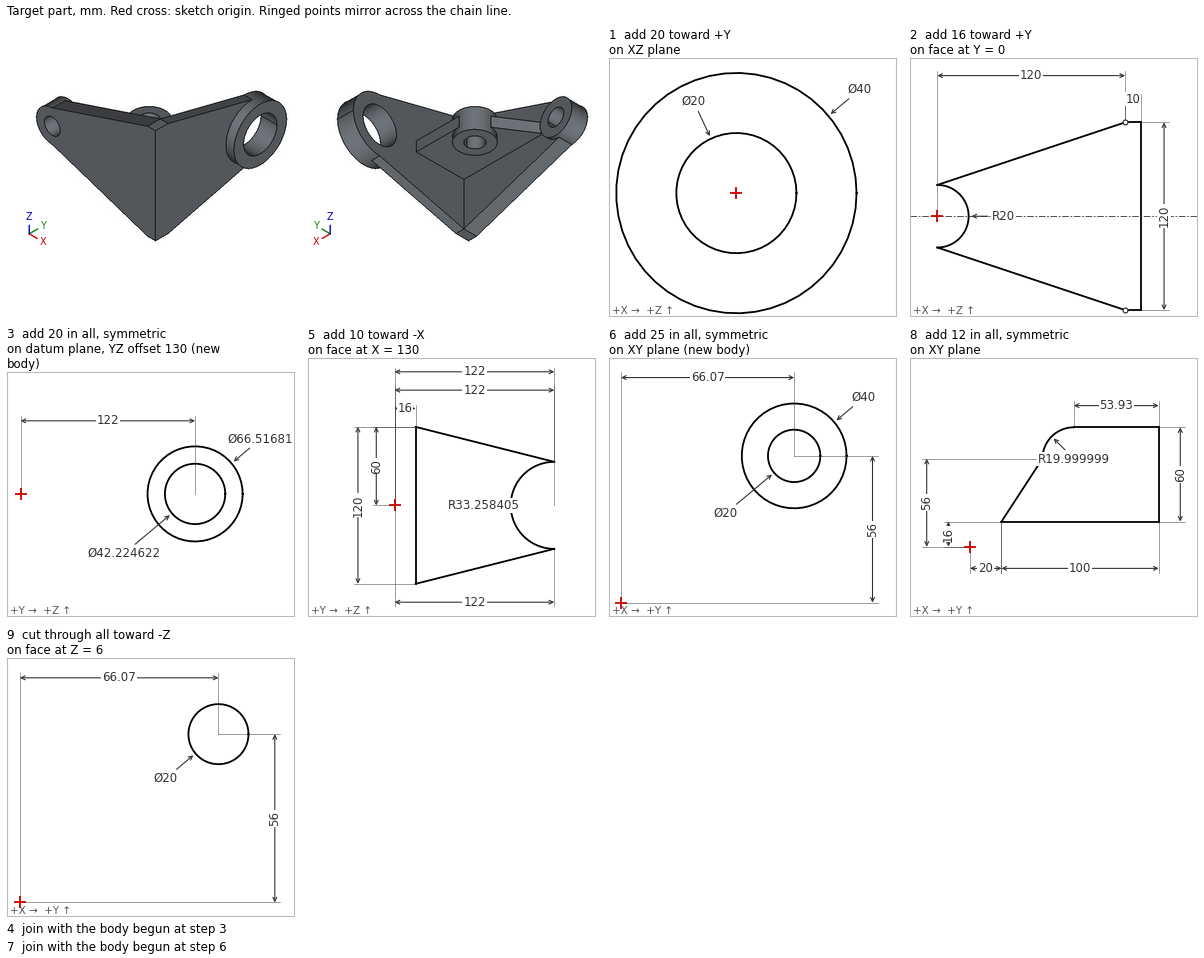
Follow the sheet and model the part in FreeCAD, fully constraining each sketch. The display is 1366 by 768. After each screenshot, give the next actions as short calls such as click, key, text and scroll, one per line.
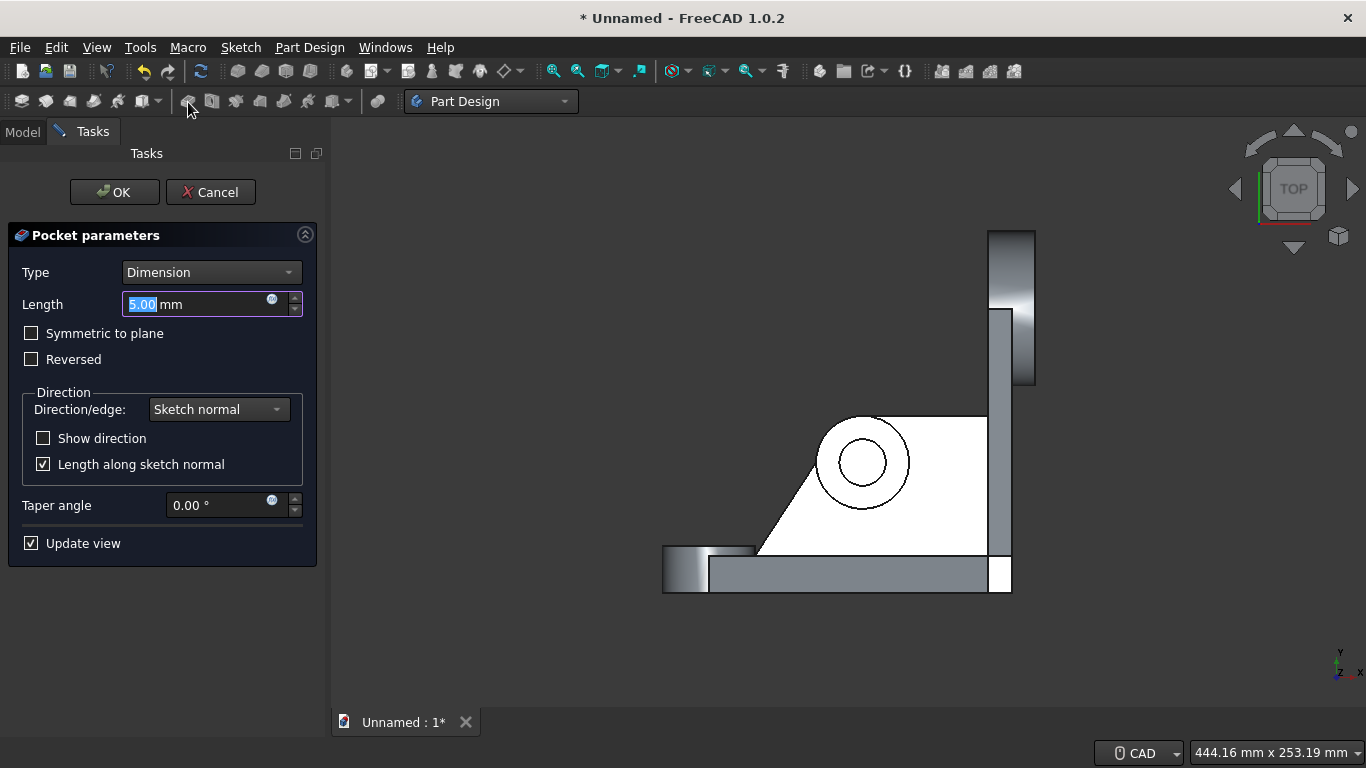
click(212, 272)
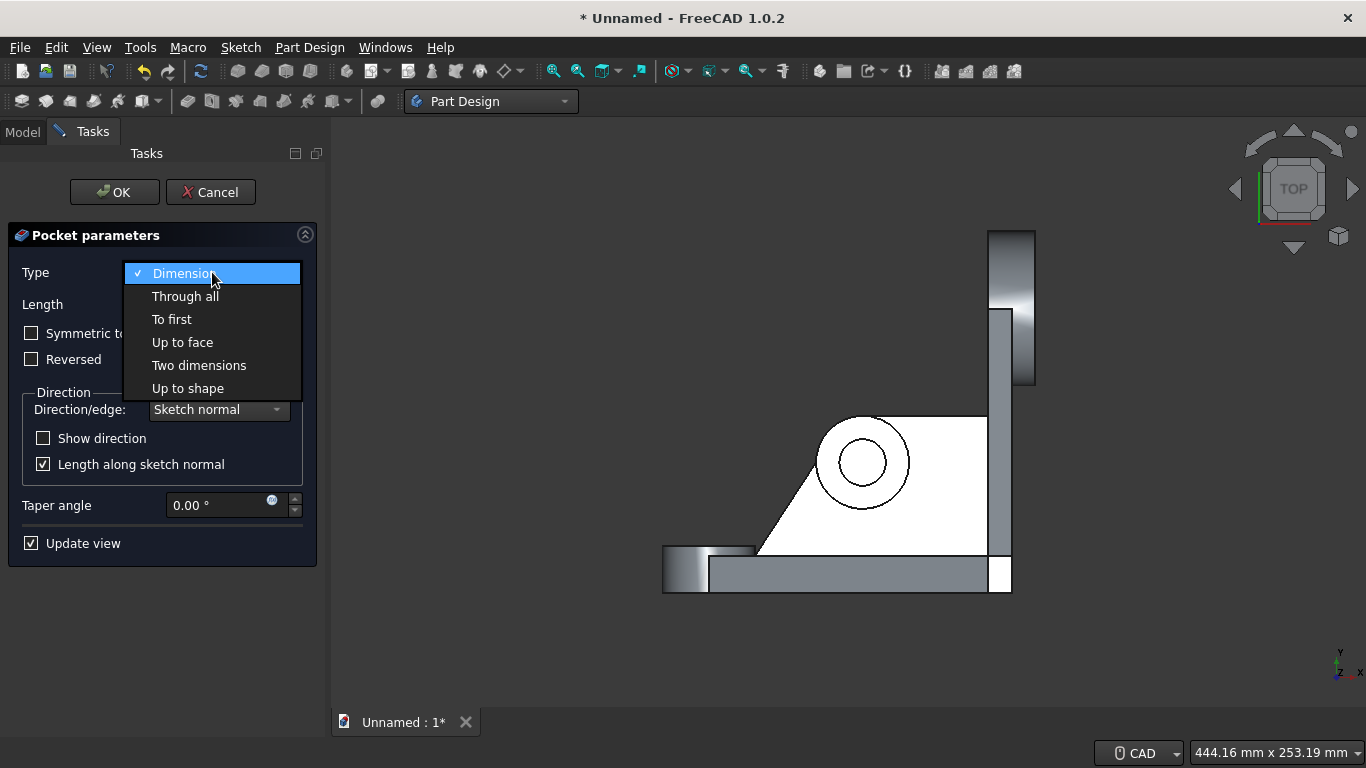
click(212, 296)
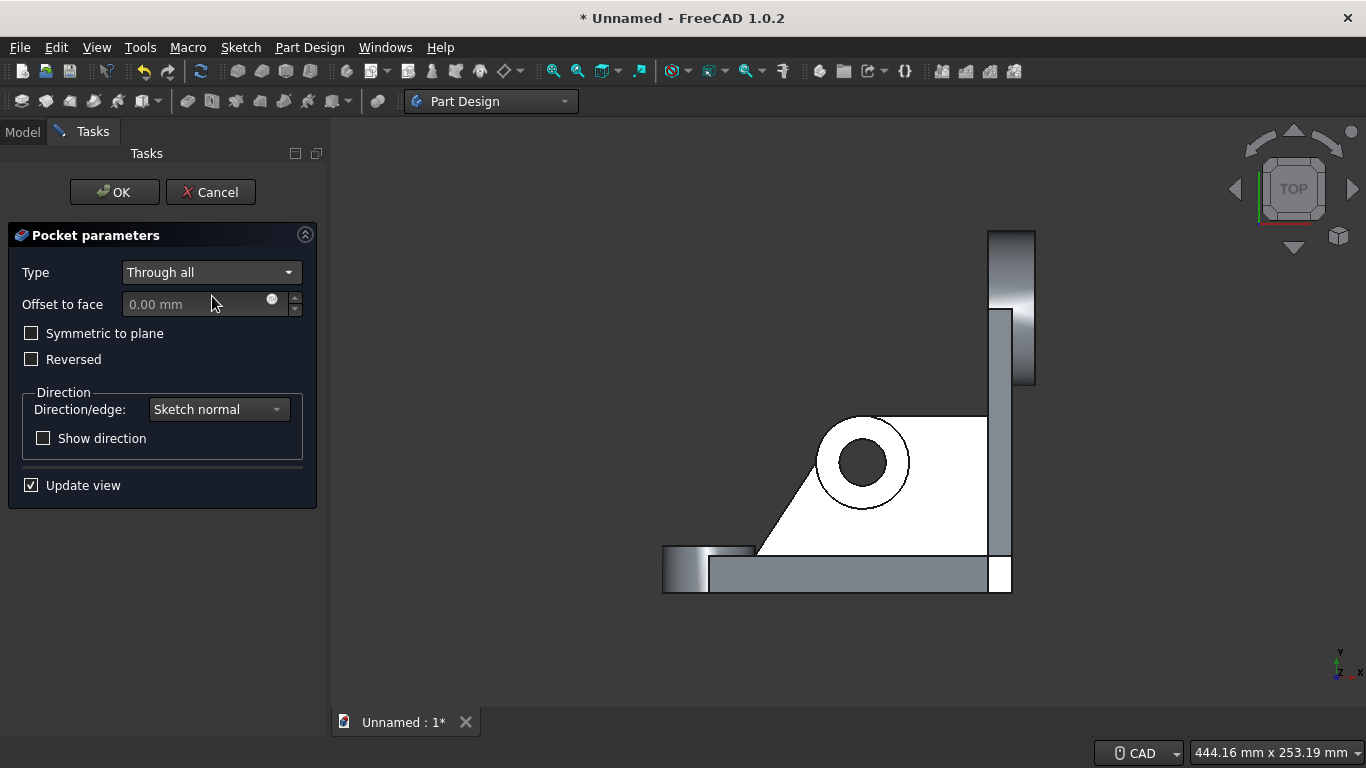
click(115, 192)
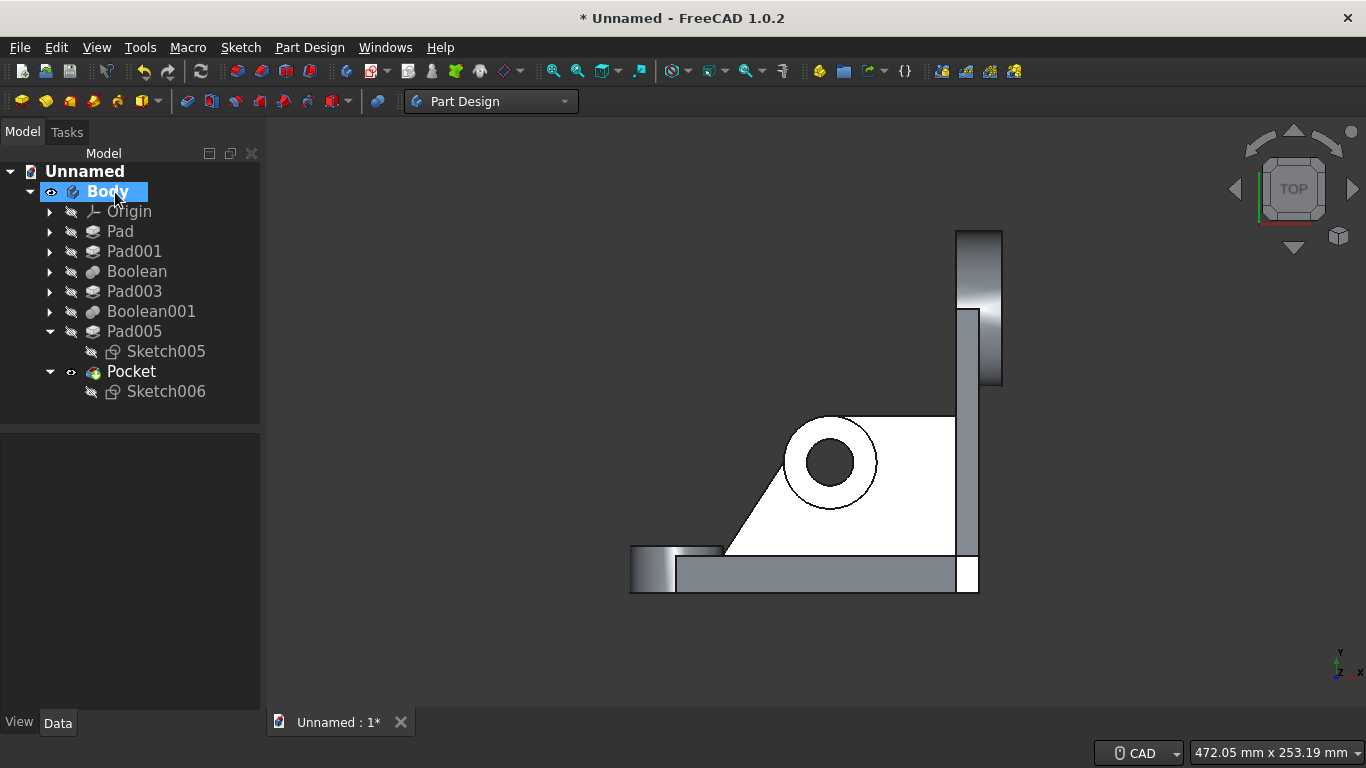
key(0)